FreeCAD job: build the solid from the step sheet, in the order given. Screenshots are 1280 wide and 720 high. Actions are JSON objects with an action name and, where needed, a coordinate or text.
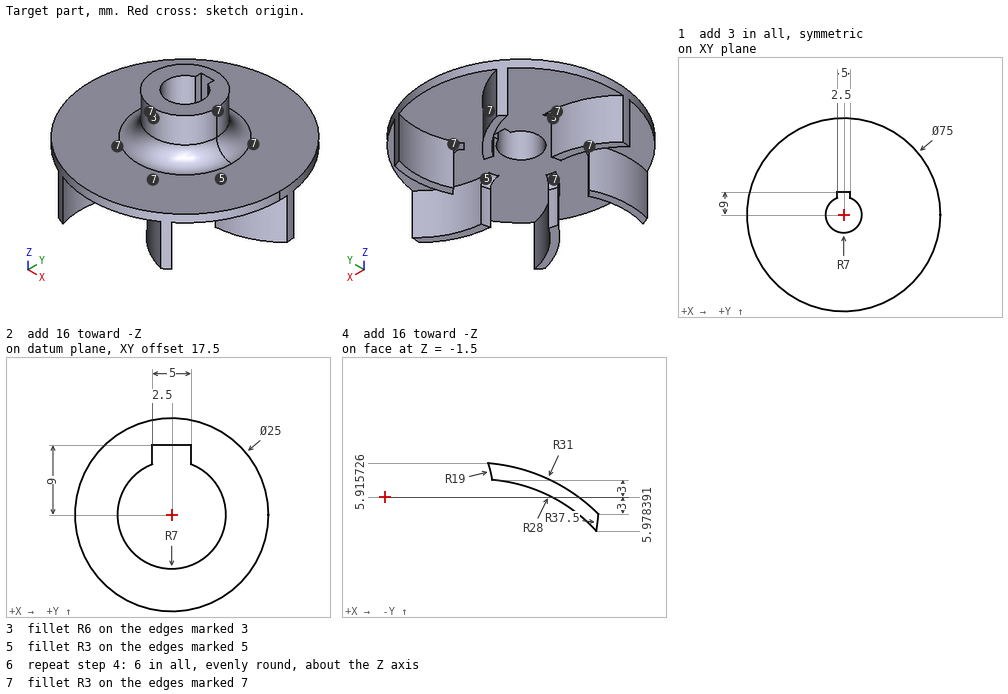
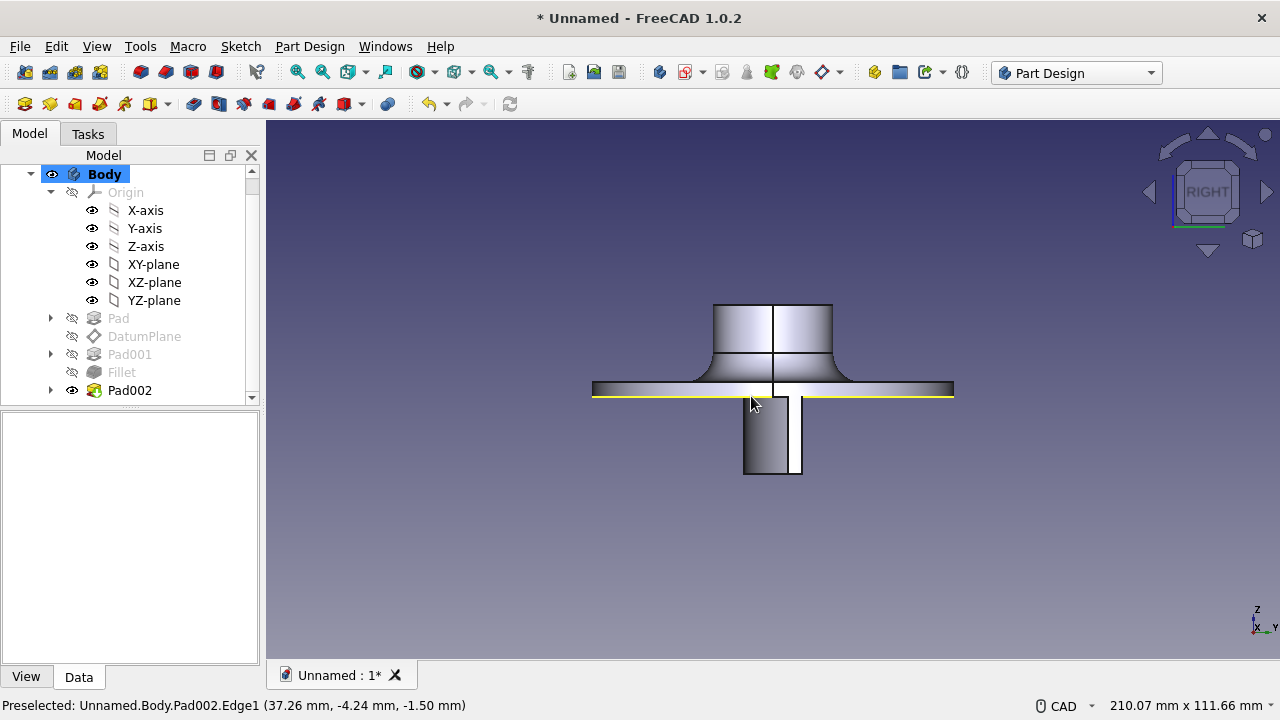
{"action": "key", "text": "5"}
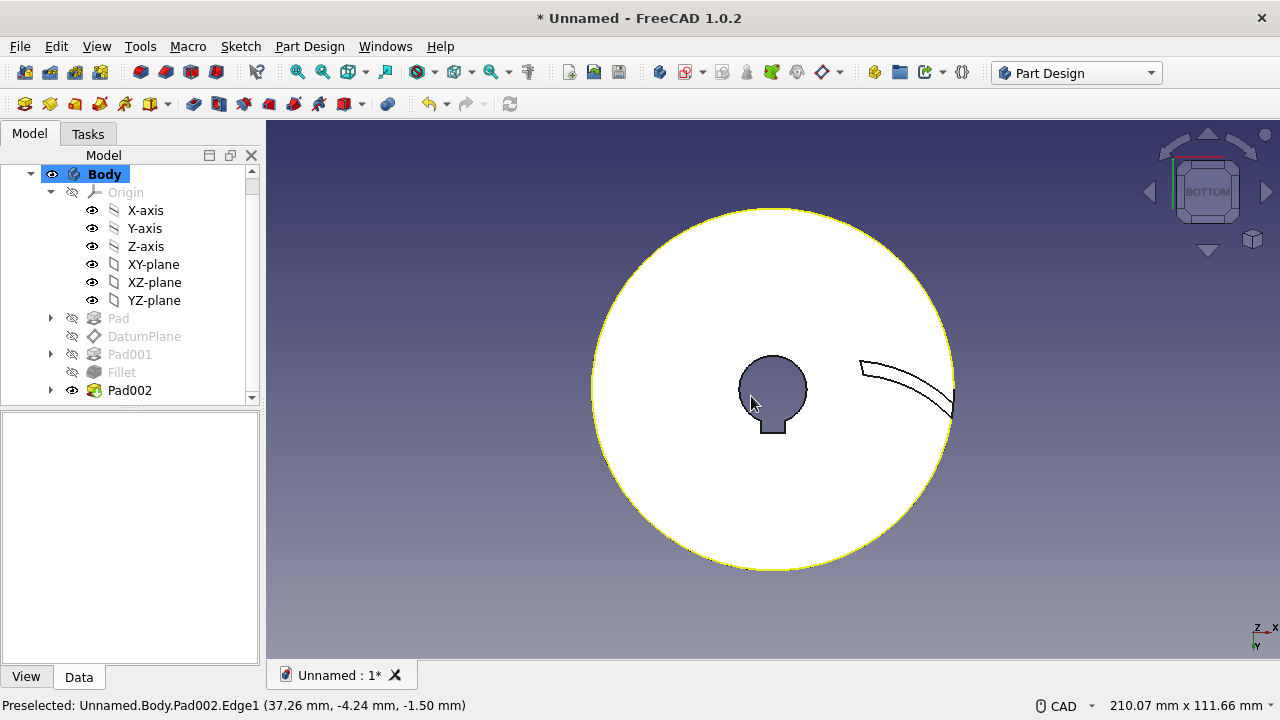
{"action": "scroll", "coordinate": [862, 367], "scroll_direction": "up", "scroll_amount": 6}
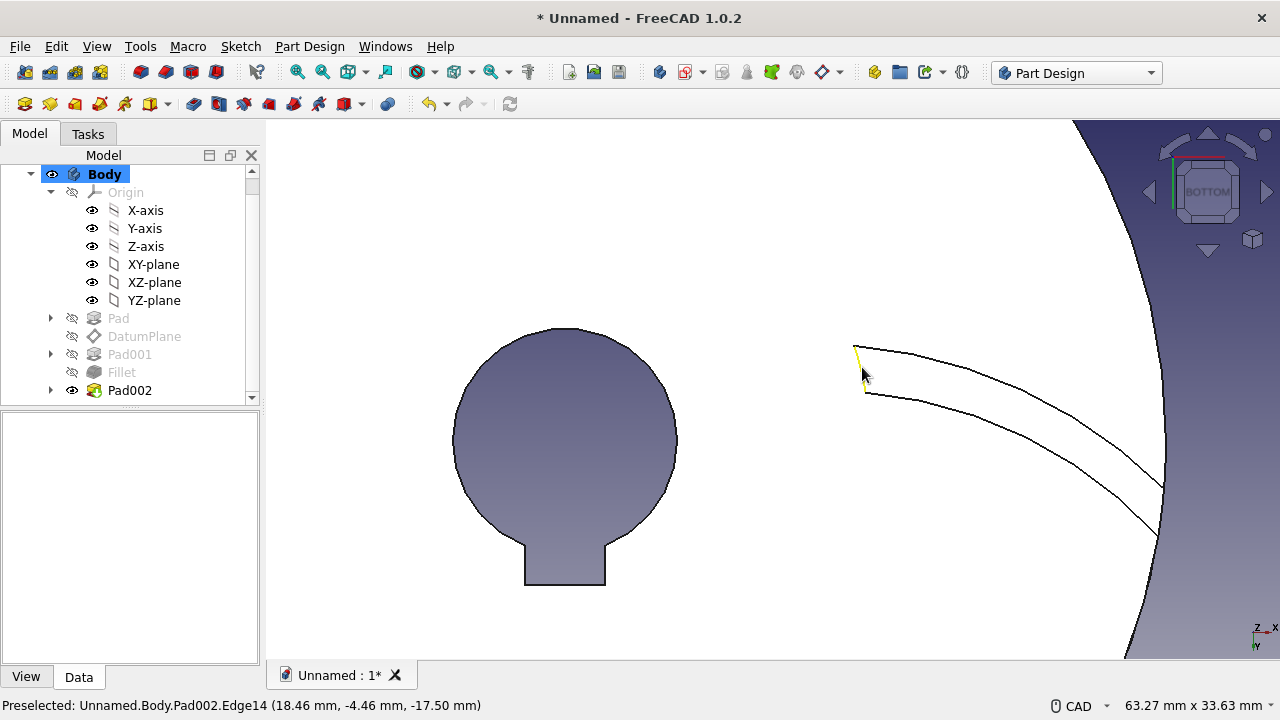
{"action": "left_click", "coordinate": [298, 72]}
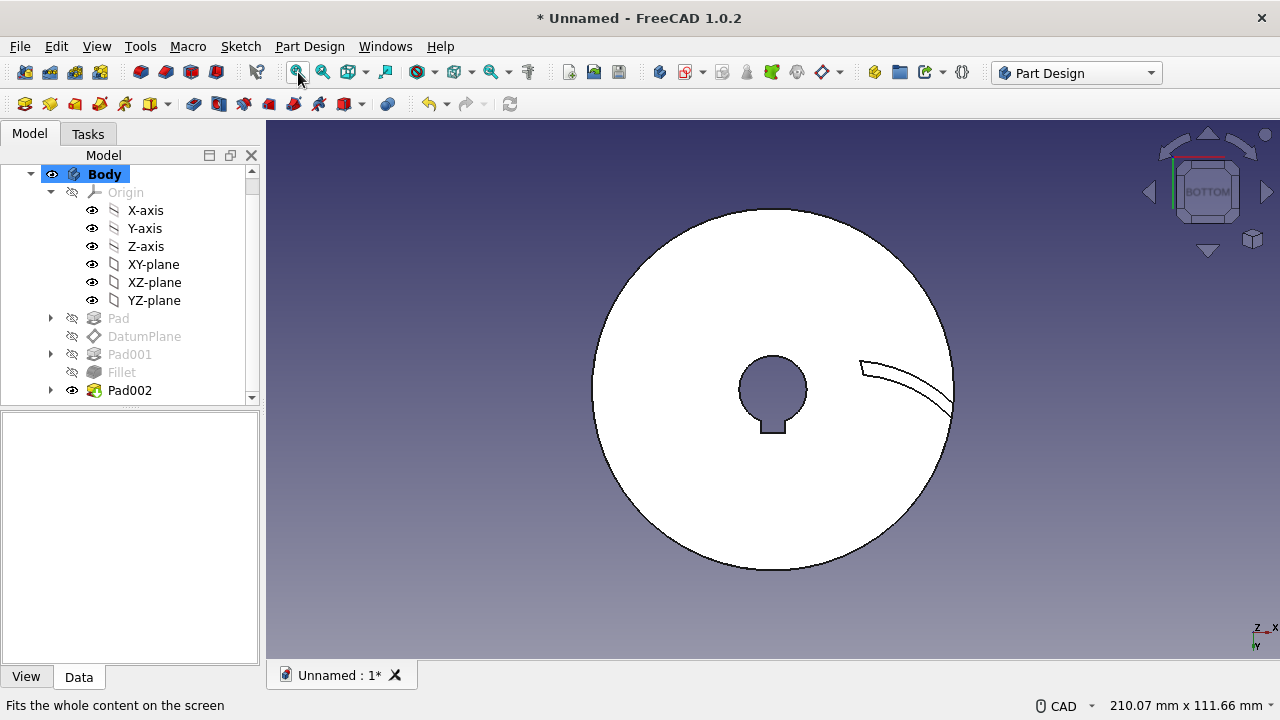
{"action": "key", "text": "4"}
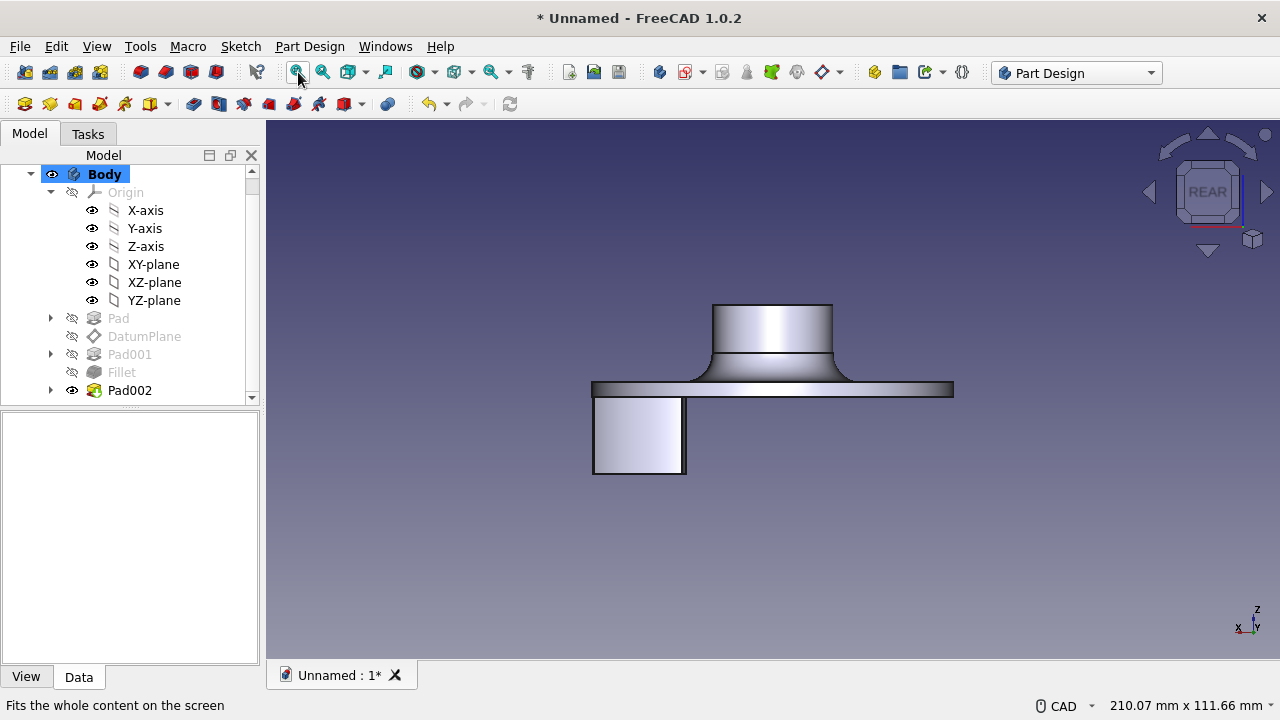
{"action": "left_click", "coordinate": [298, 72]}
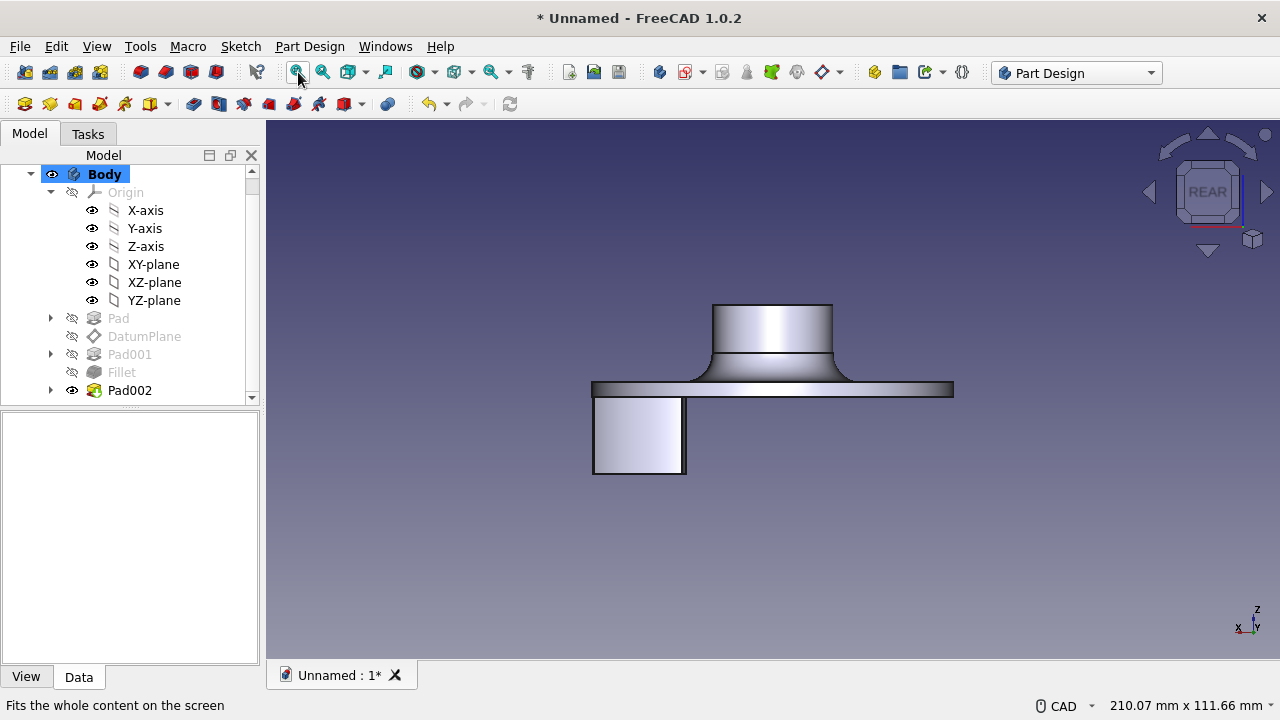
{"action": "scroll", "coordinate": [684, 396], "scroll_direction": "up", "scroll_amount": 6}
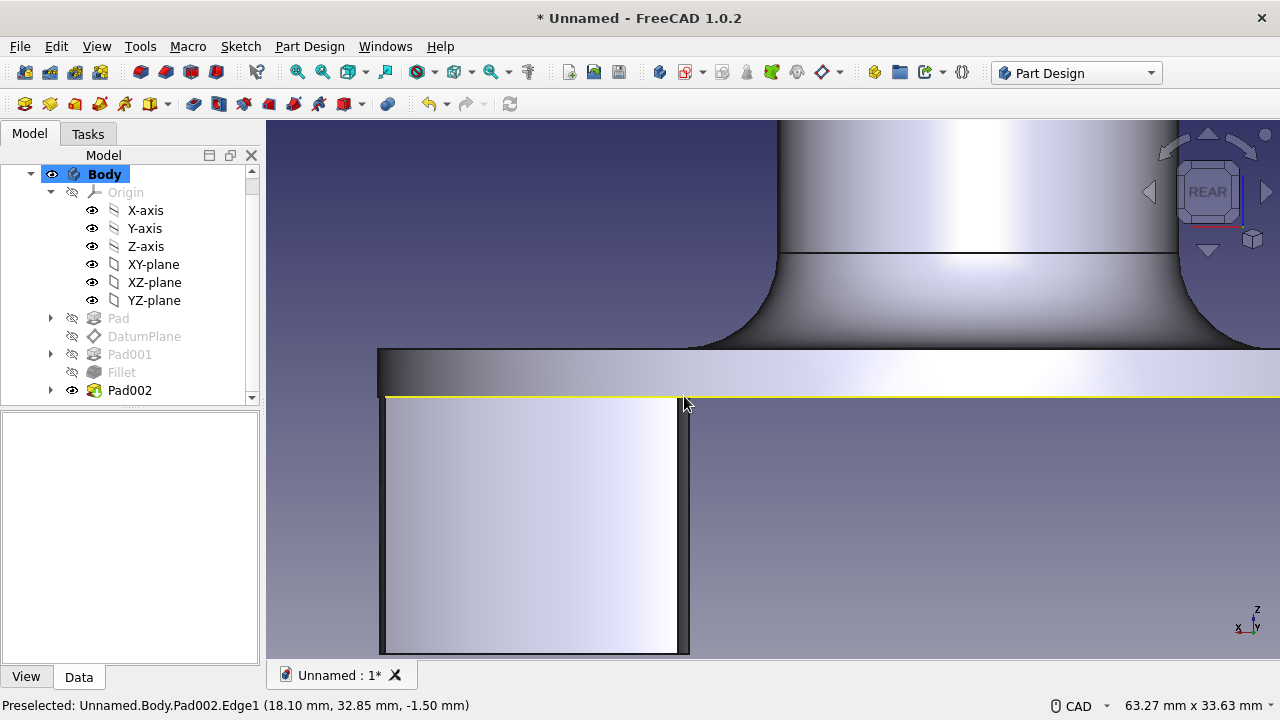
{"action": "left_click", "coordinate": [298, 72]}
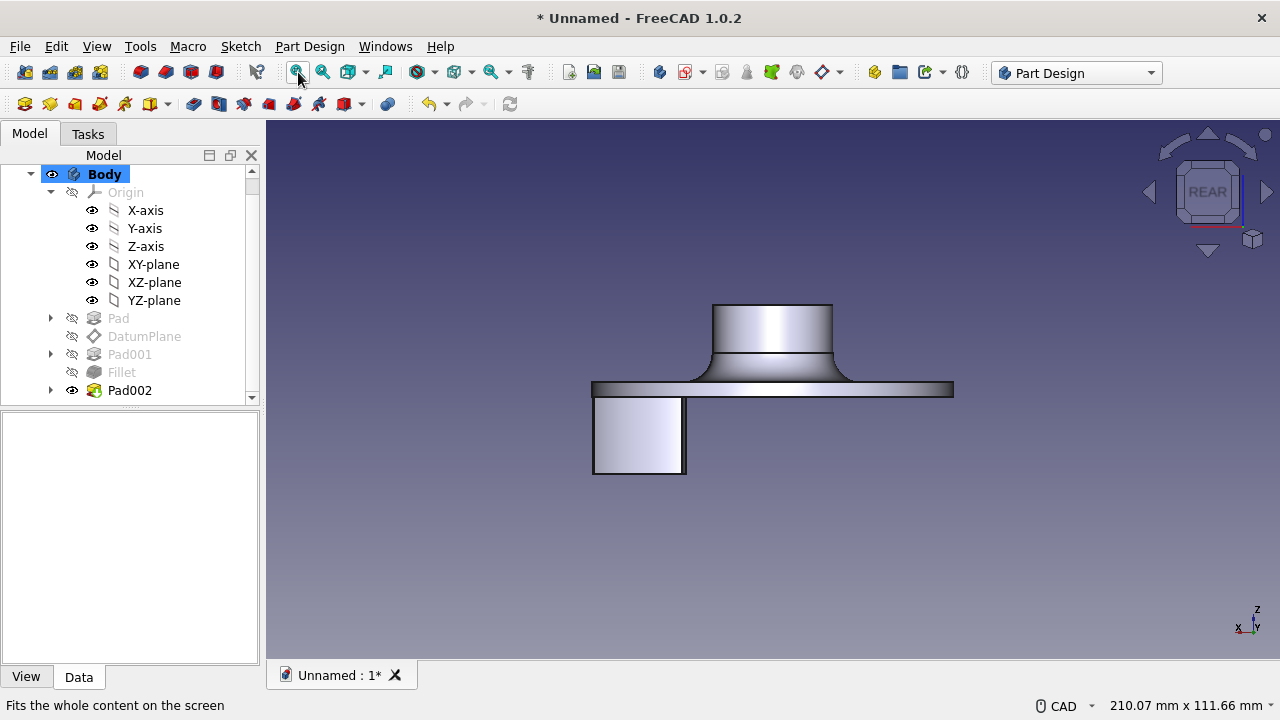
{"action": "key", "text": "6"}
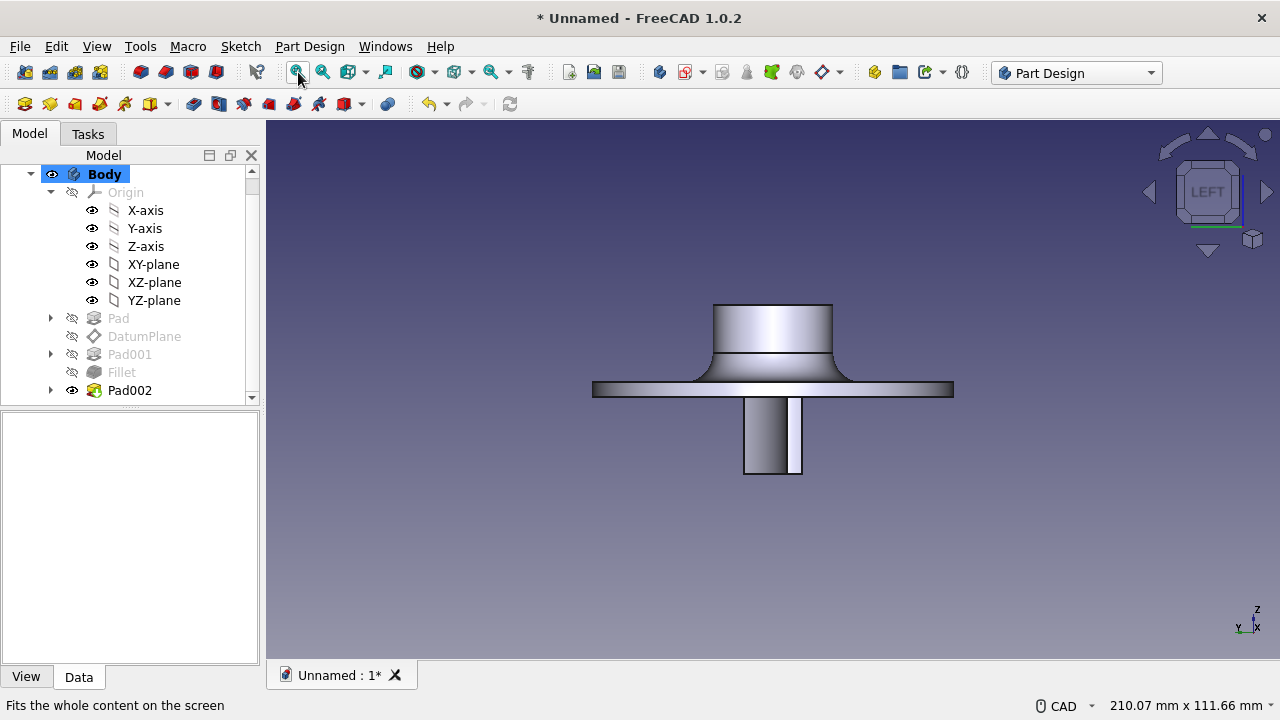
{"action": "left_click", "coordinate": [298, 72]}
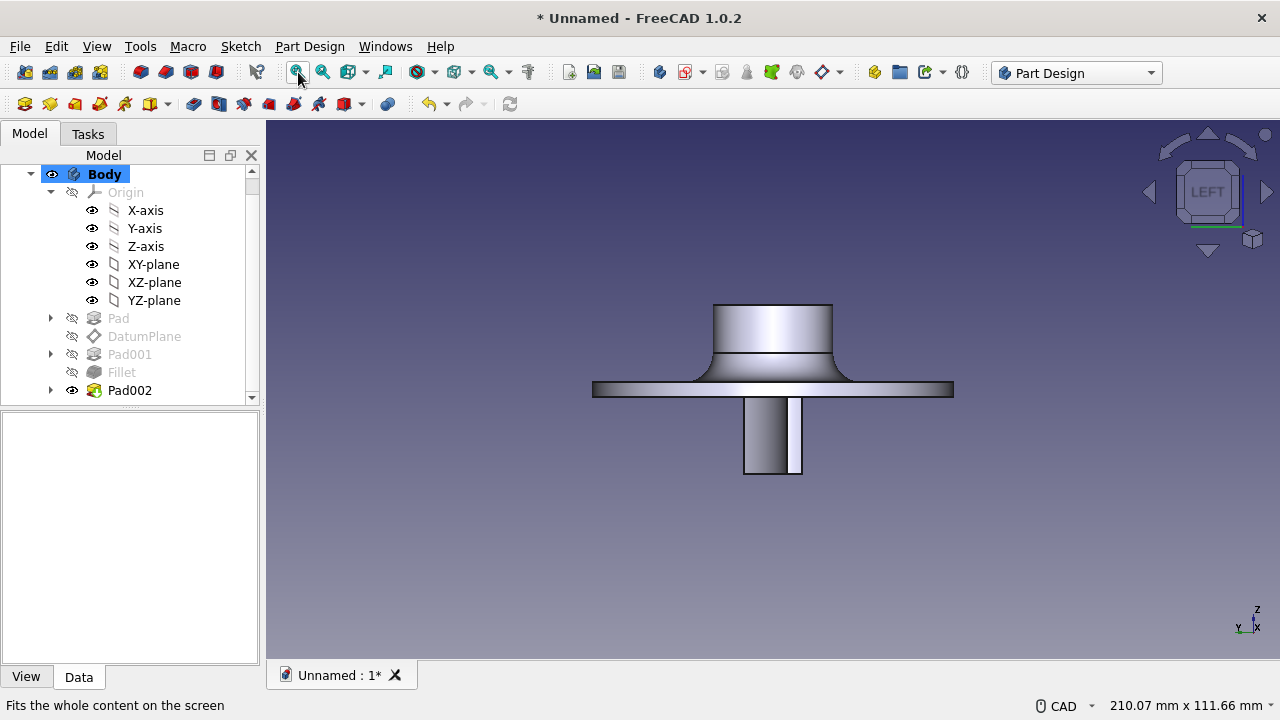
{"action": "scroll", "coordinate": [795, 396], "scroll_direction": "up", "scroll_amount": 6}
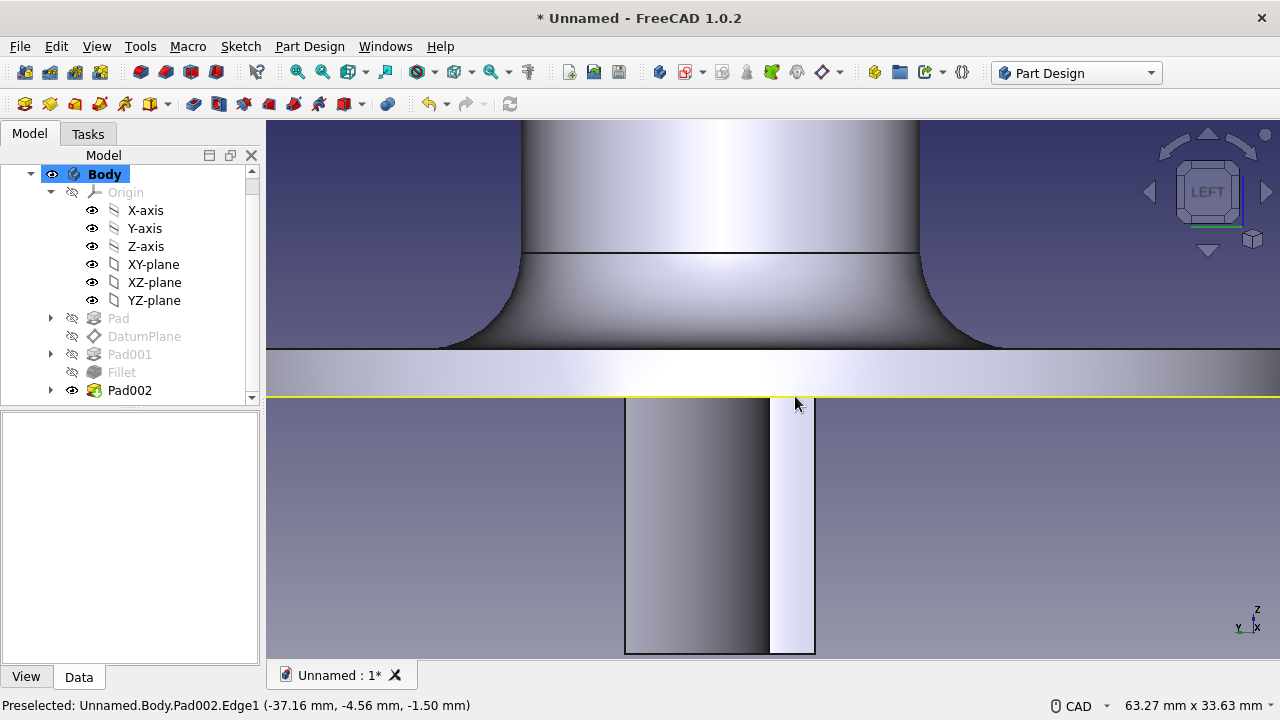
{"action": "left_click", "coordinate": [298, 72]}